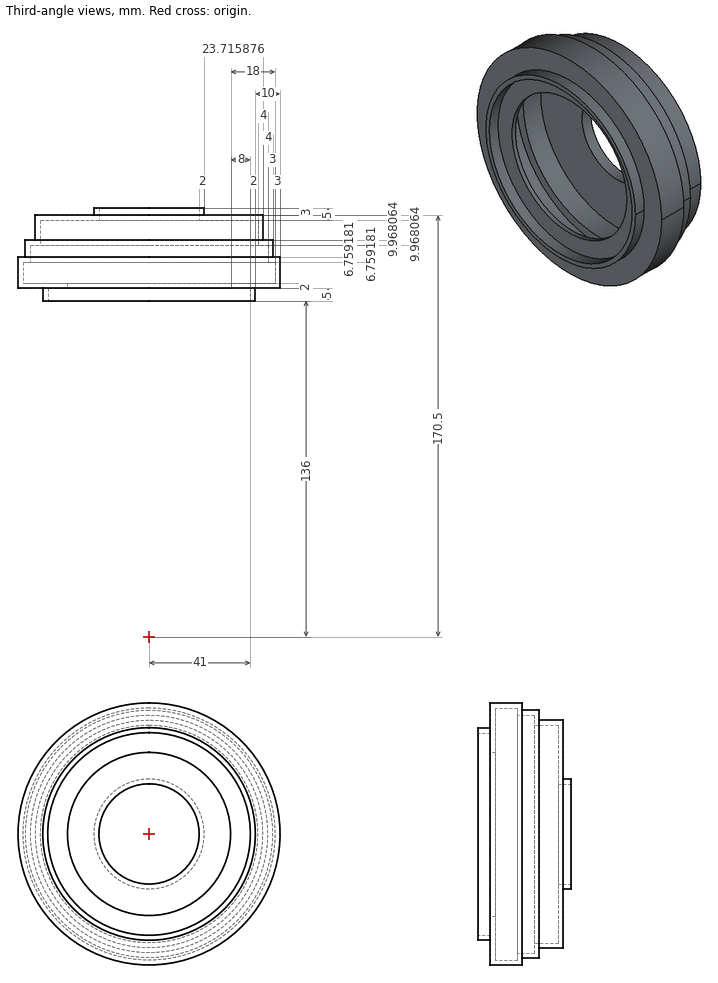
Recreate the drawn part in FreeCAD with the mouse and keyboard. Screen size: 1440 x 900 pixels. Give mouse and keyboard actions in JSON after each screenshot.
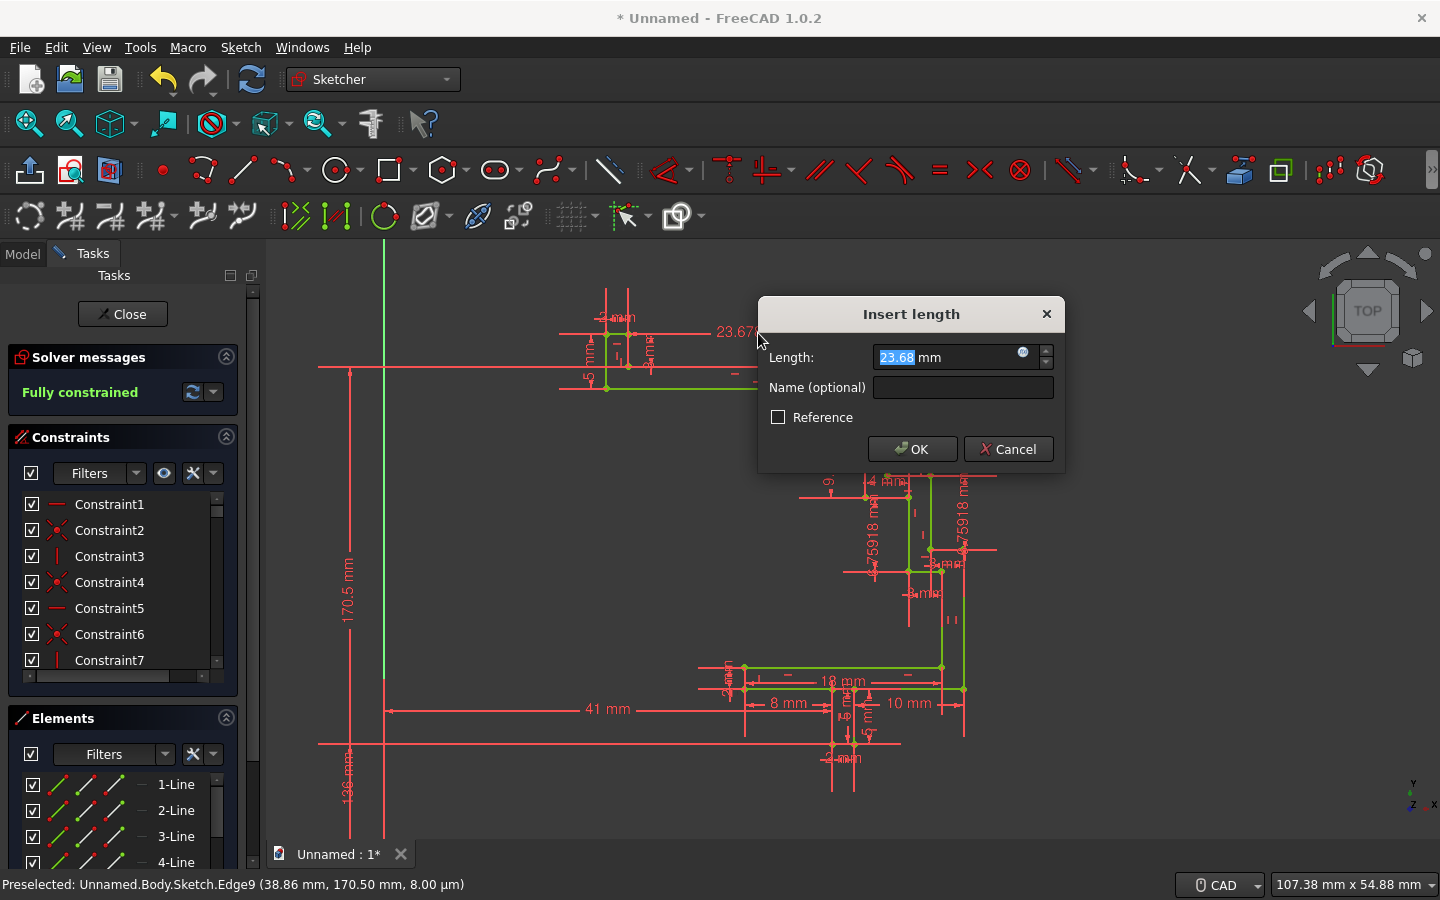
{"action": "type", "text": "23.715876"}
{"action": "key", "text": "Return"}
{"action": "key", "text": "Escape"}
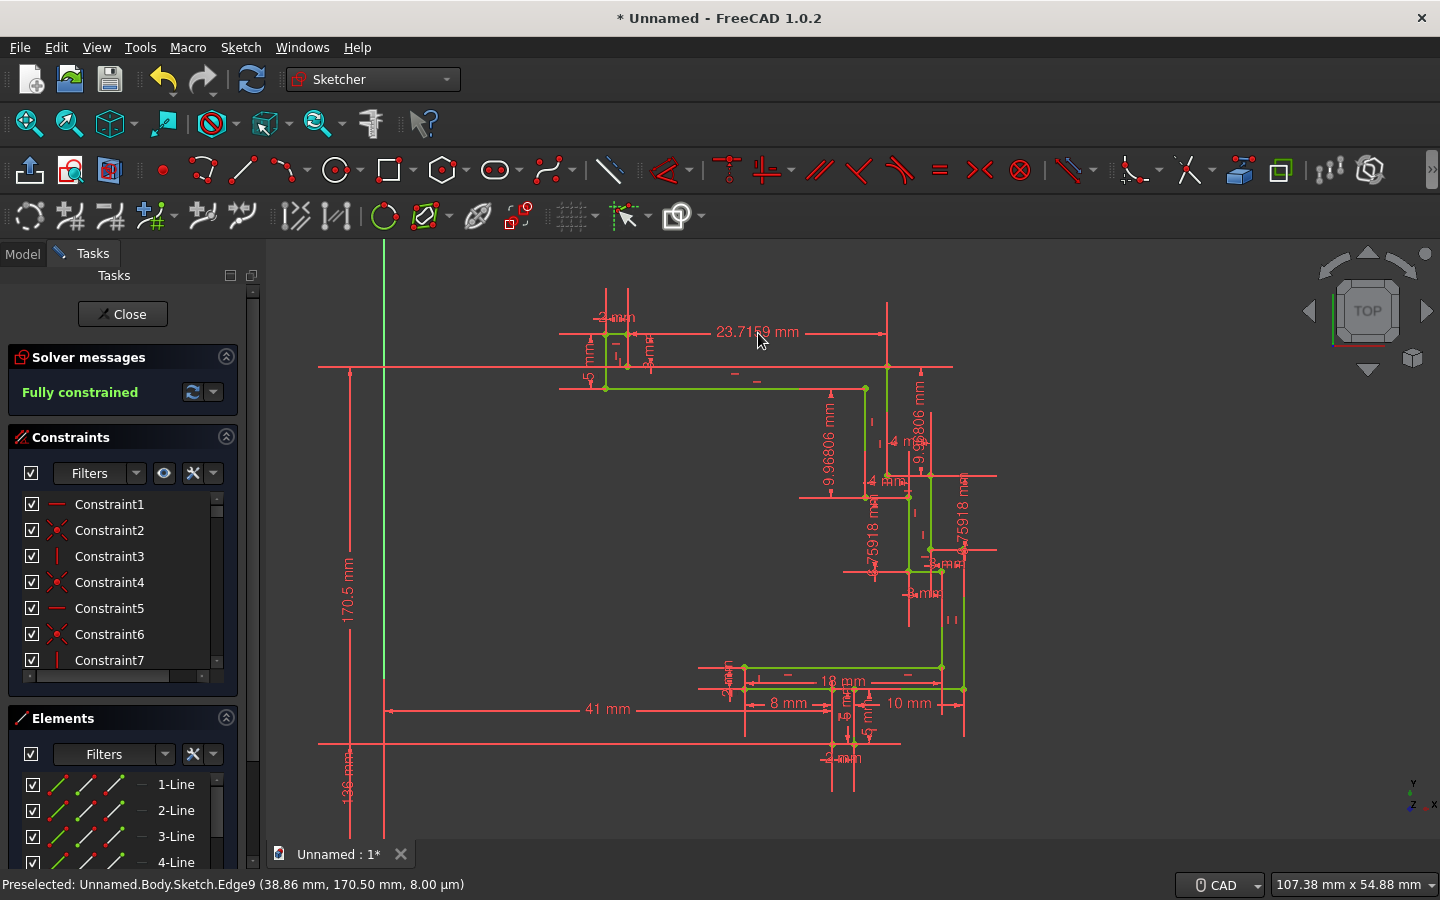
{"action": "left_click", "coordinate": [123, 314]}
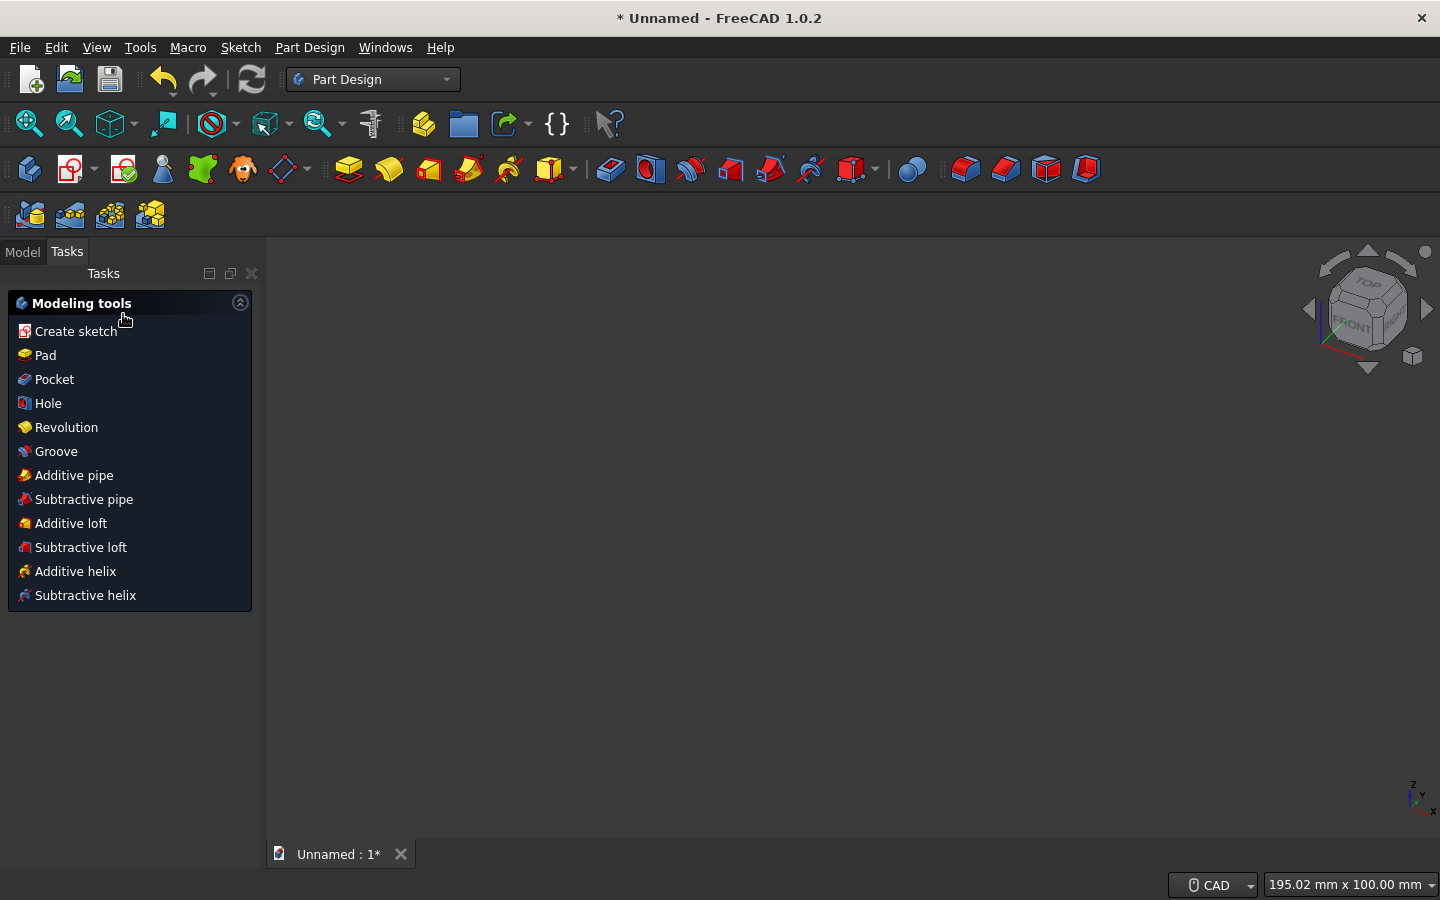
{"action": "left_click", "coordinate": [390, 170]}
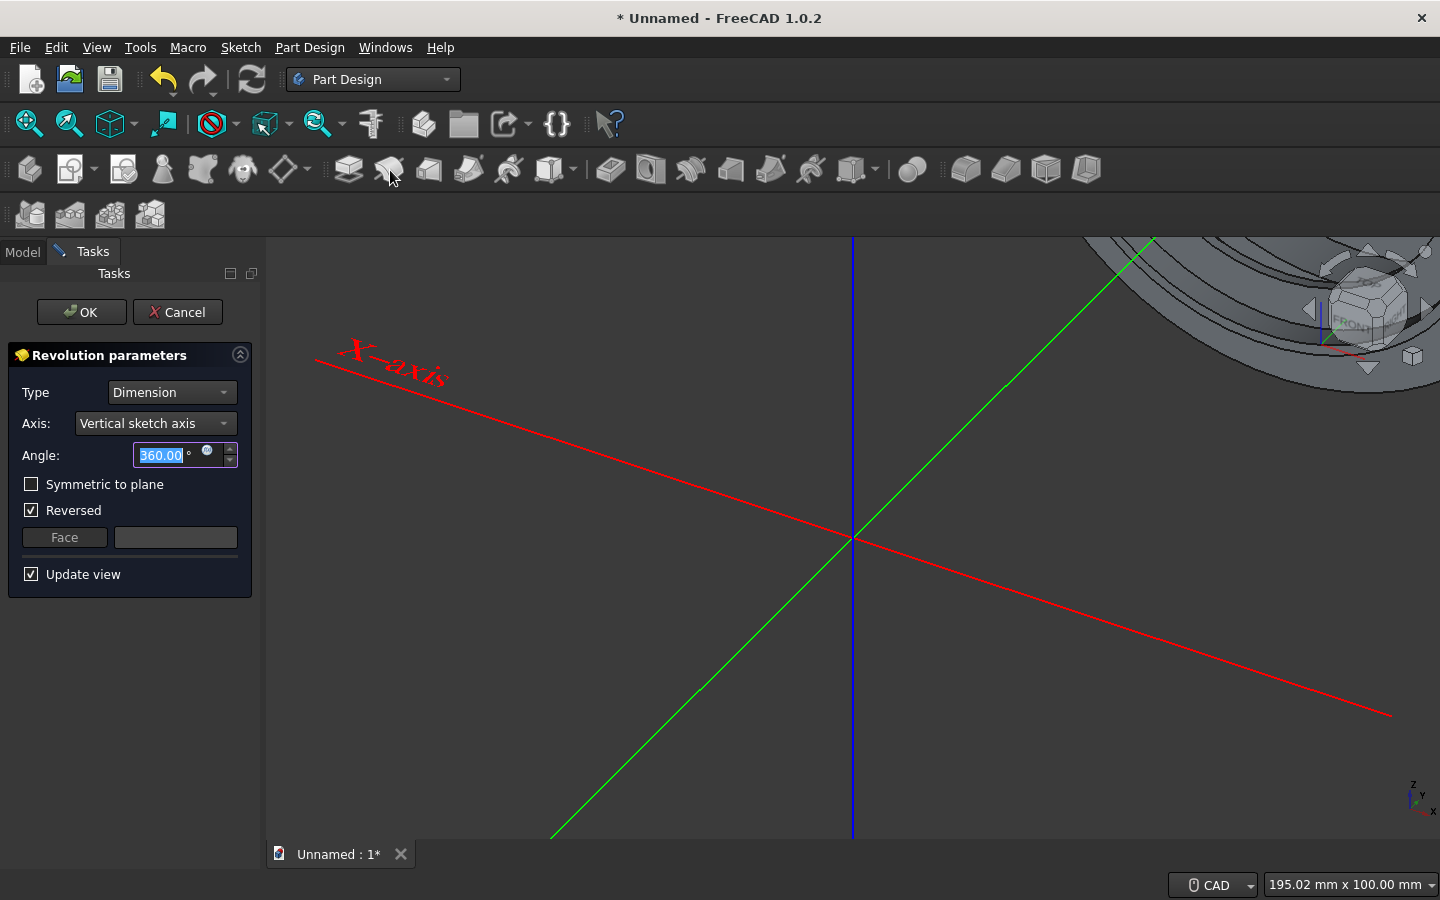
{"action": "left_click", "coordinate": [82, 312]}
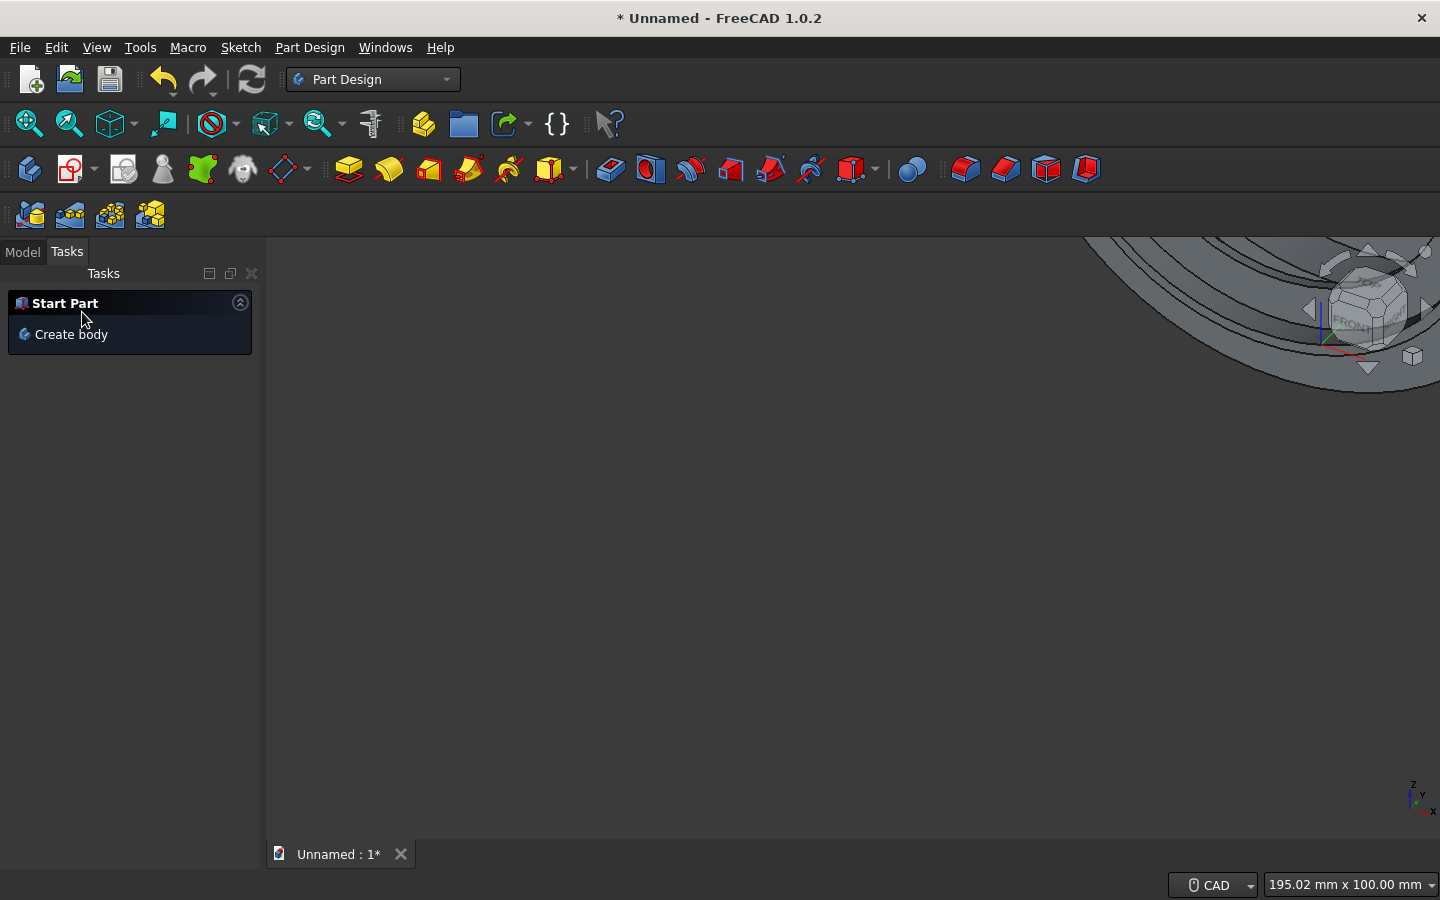
{"action": "key", "text": "0"}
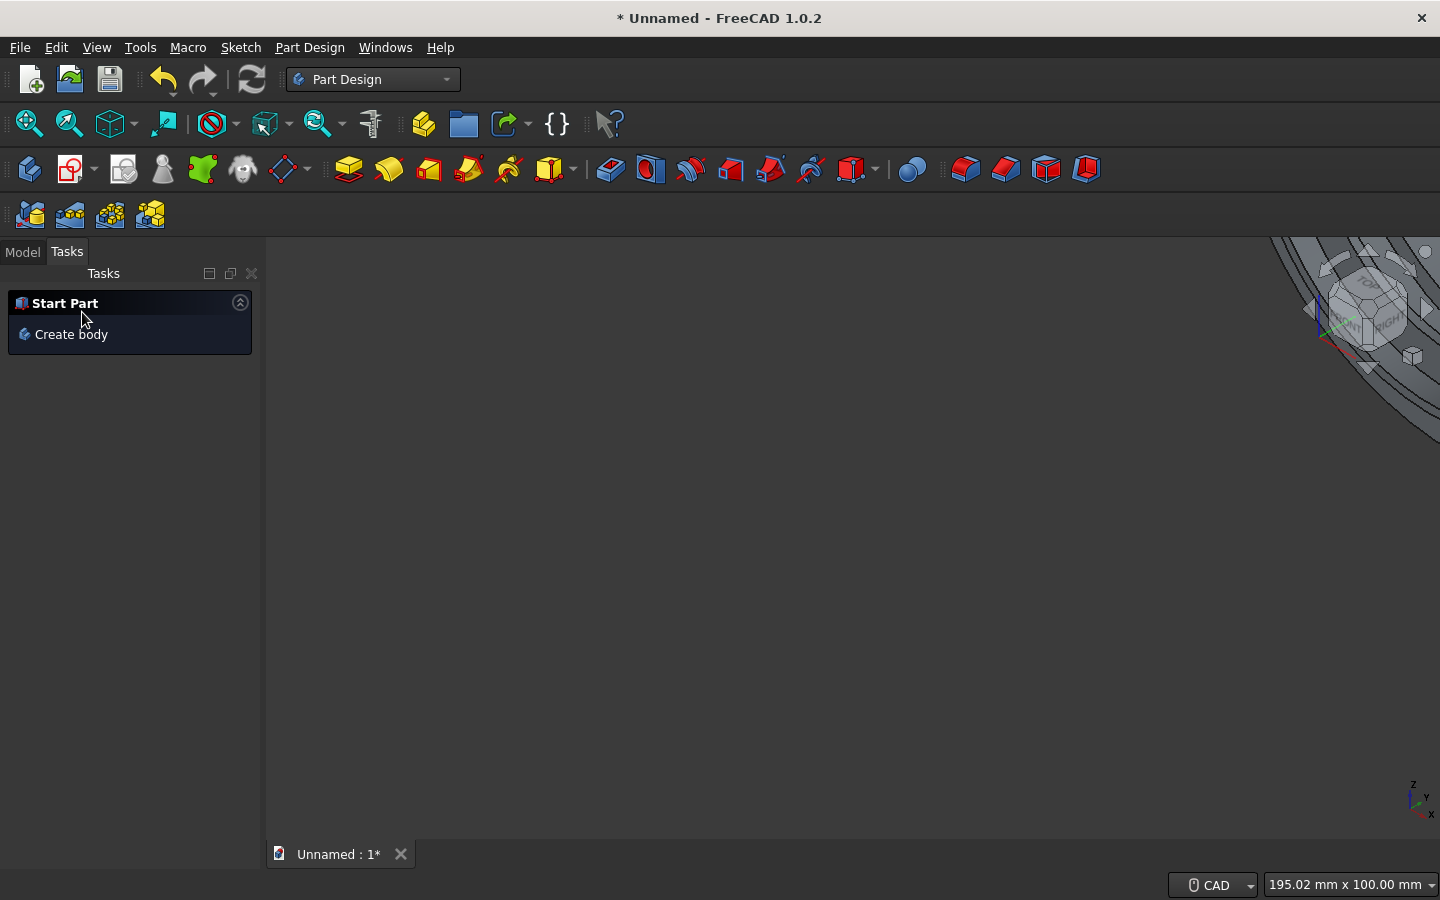
{"action": "left_click", "coordinate": [30, 124]}